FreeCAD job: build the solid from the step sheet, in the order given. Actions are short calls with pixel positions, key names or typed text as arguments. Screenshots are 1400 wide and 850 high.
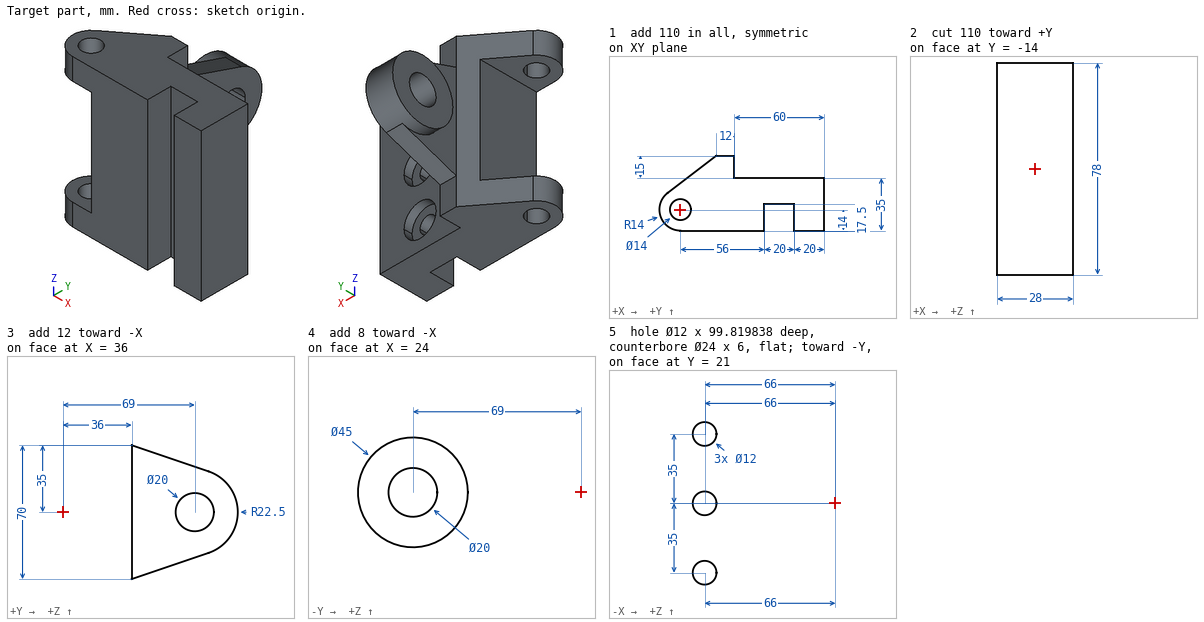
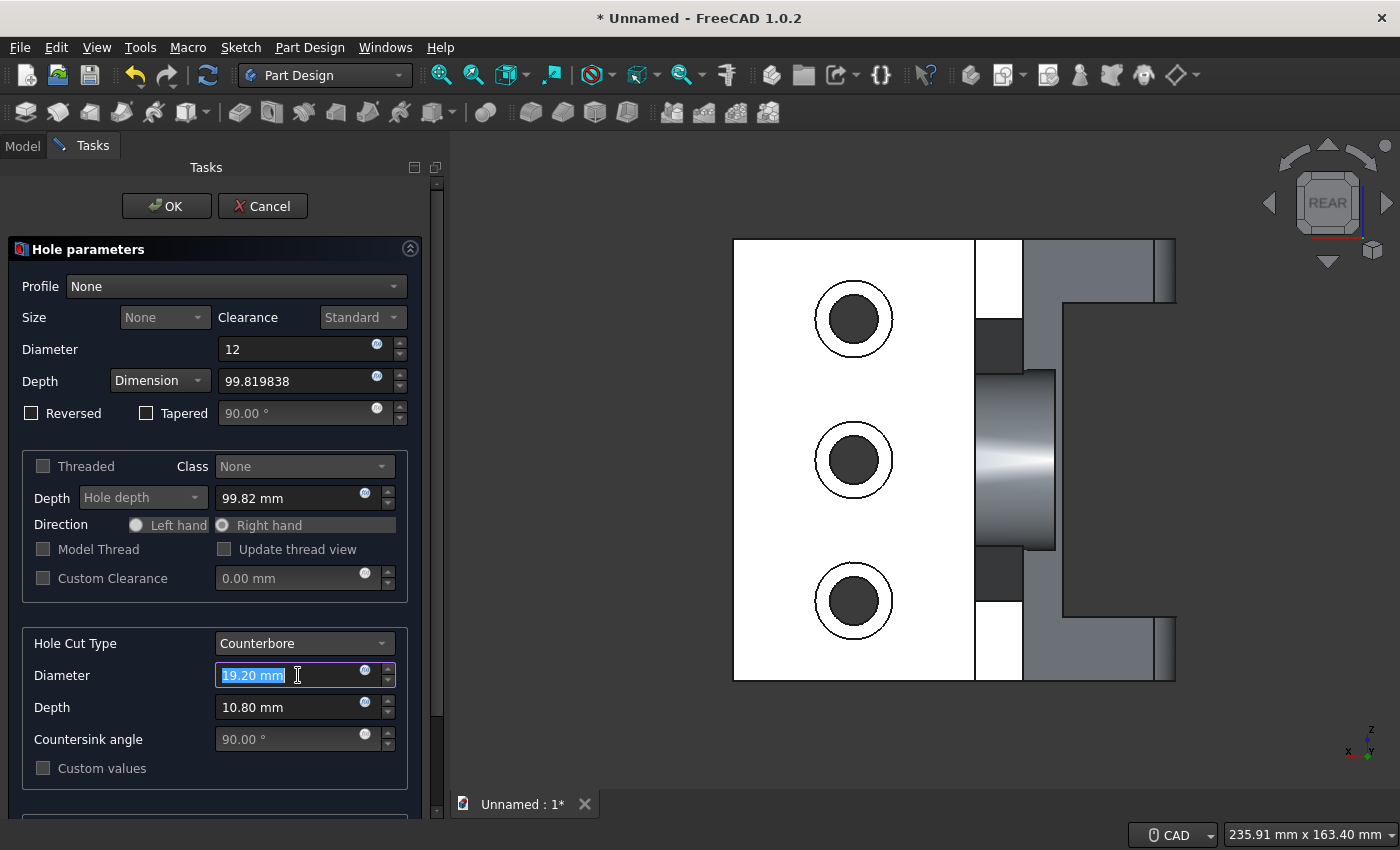
text(24)
key(Tab)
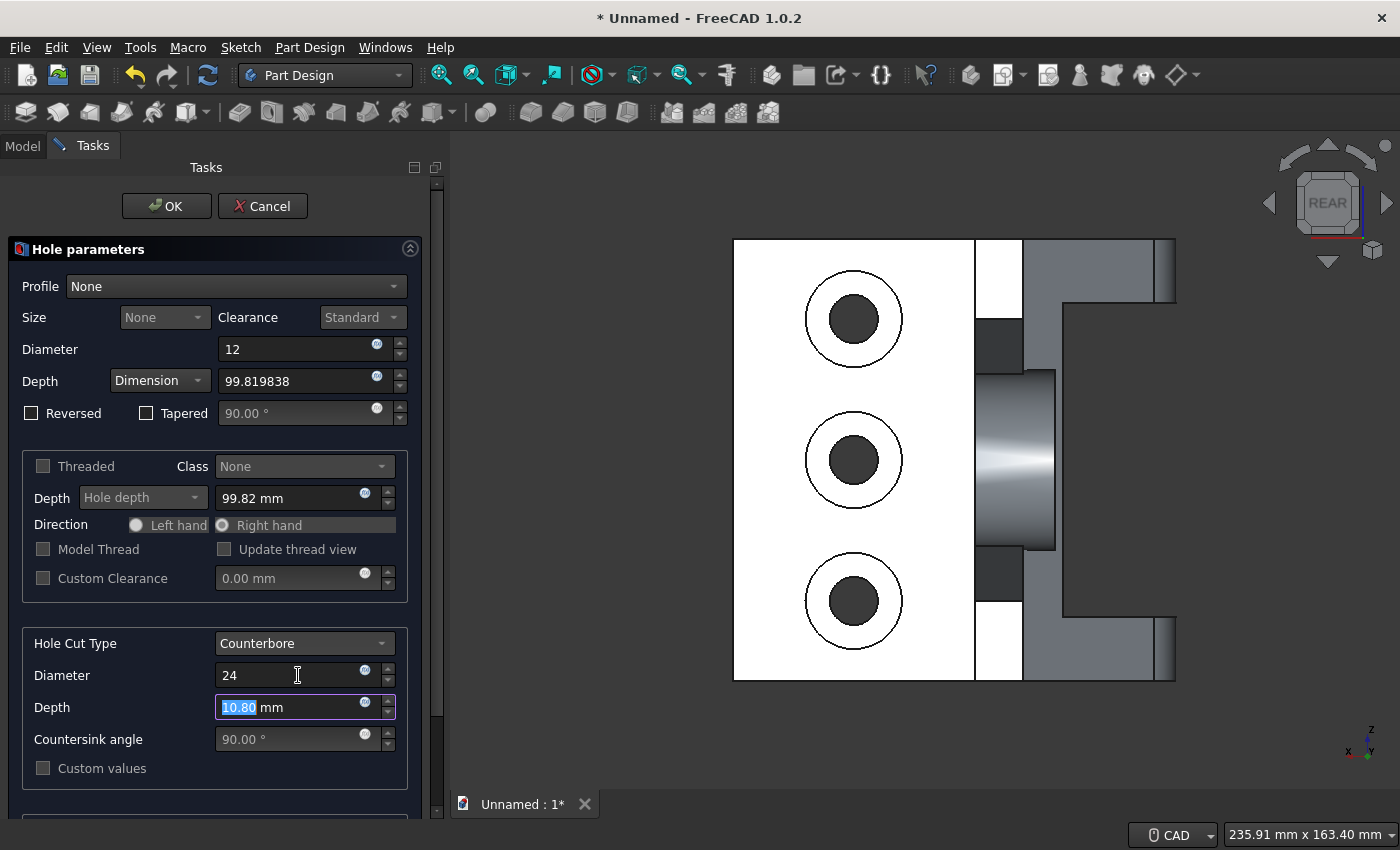
text(6)
key(Tab)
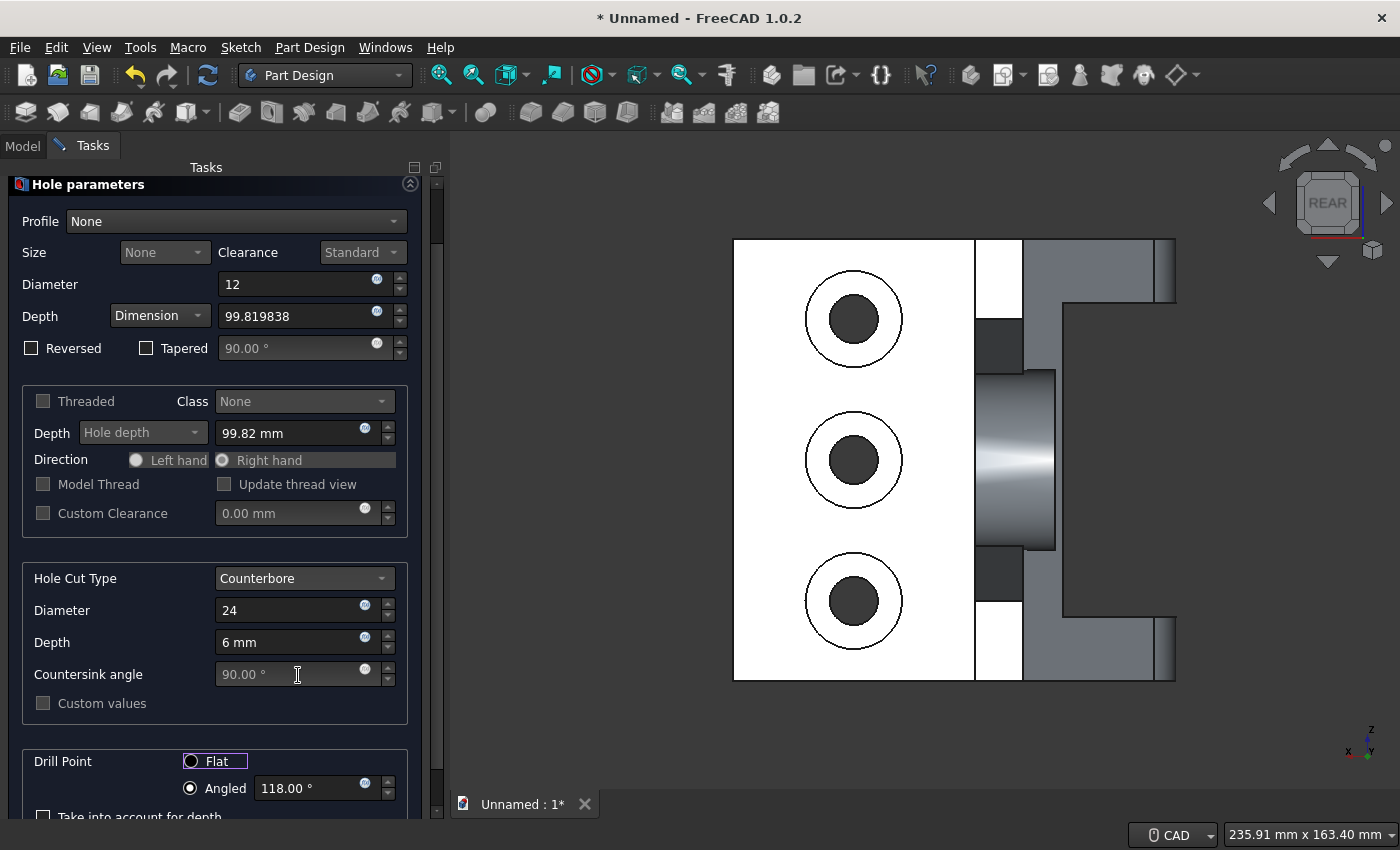
click(191, 761)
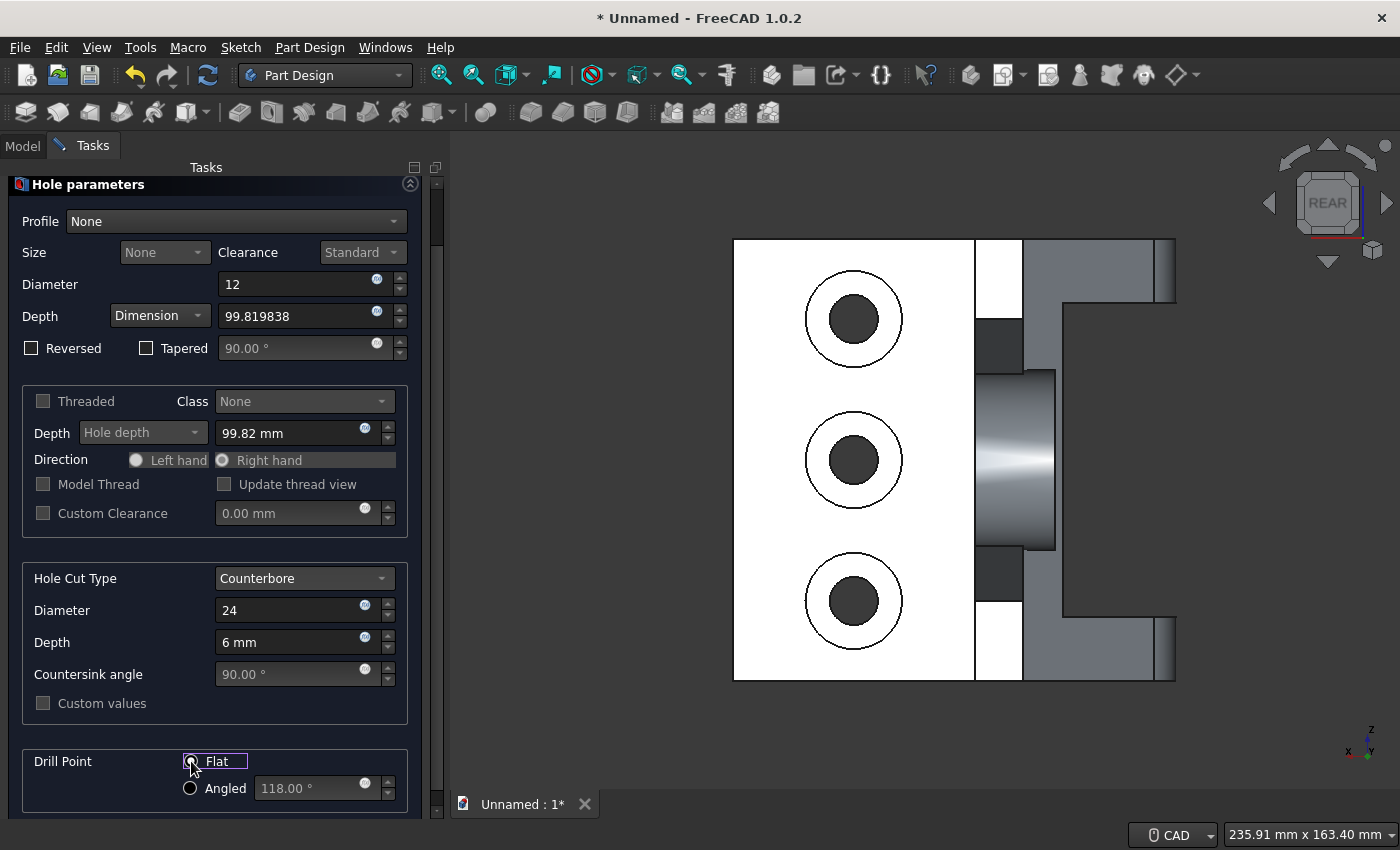
scroll(437, 498, up, 2)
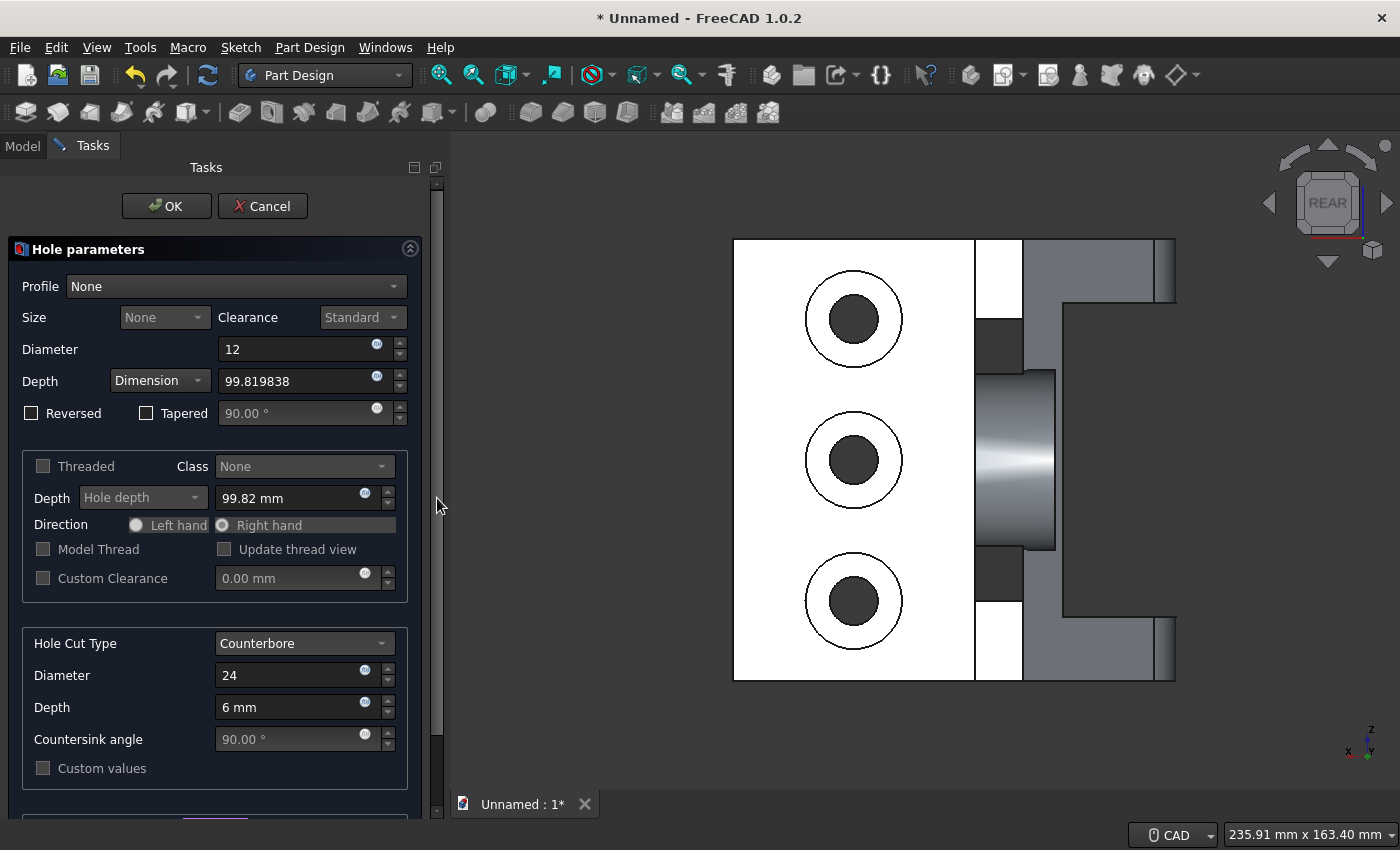
click(167, 206)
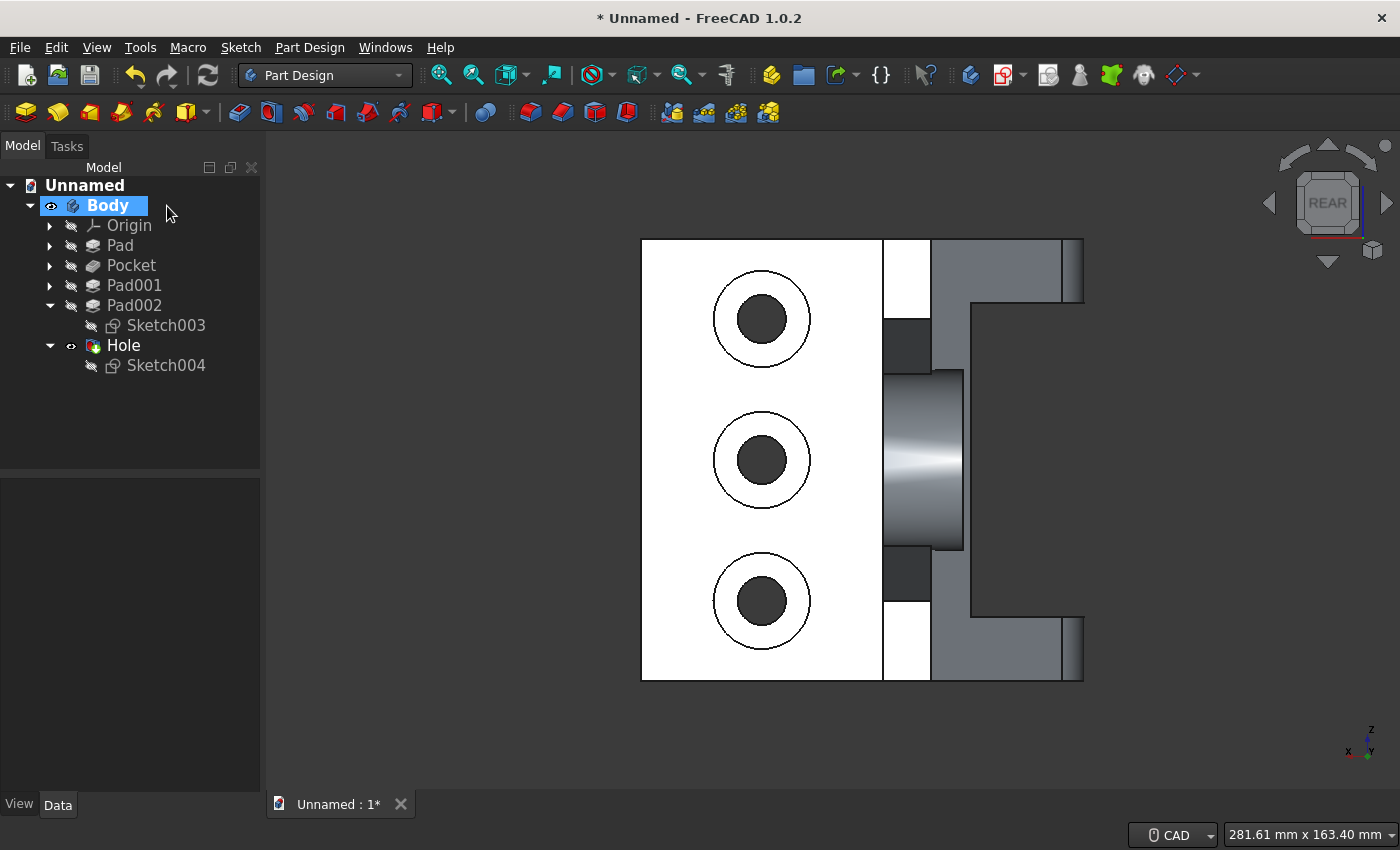
key(0)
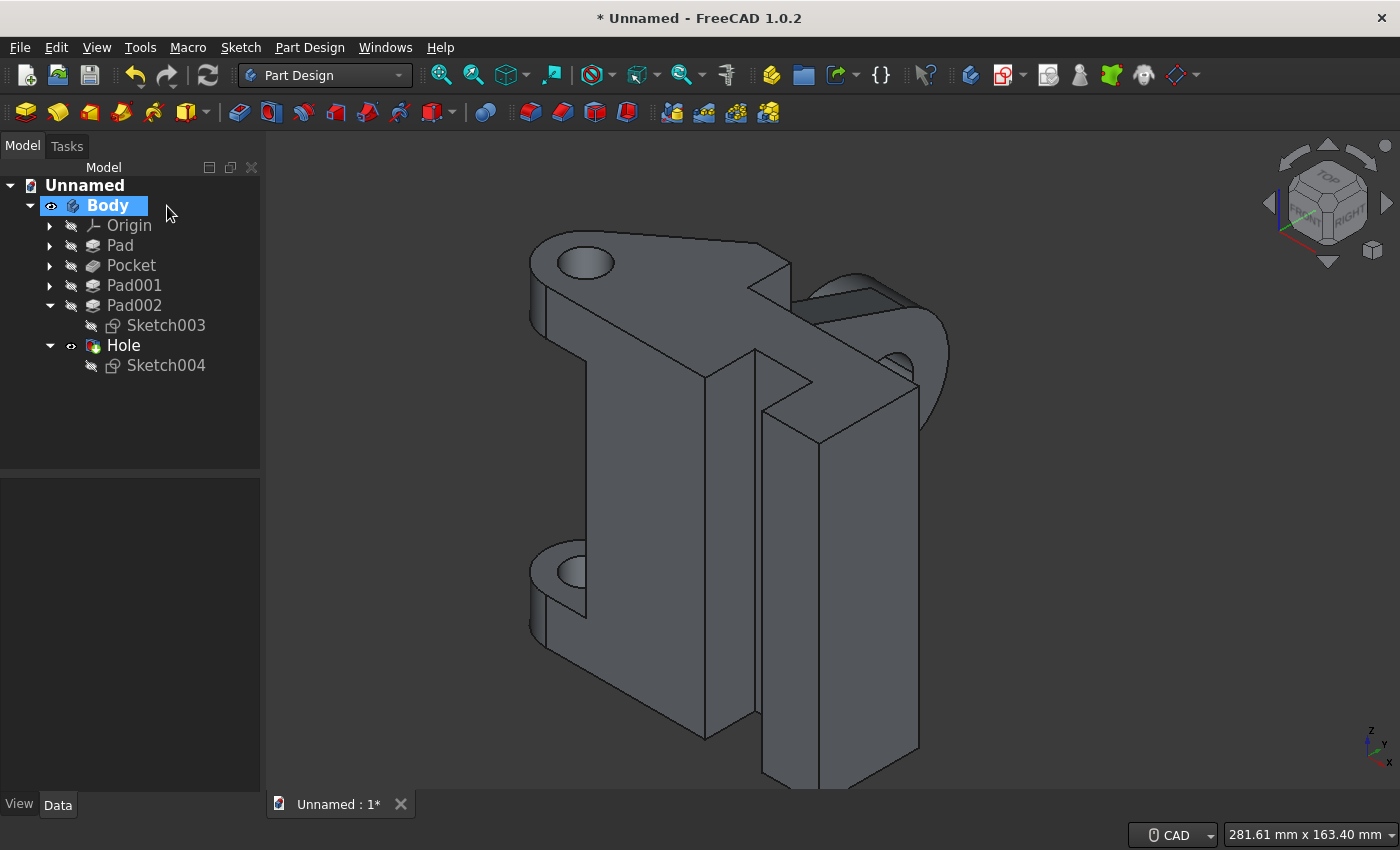
key(v)
key(f)